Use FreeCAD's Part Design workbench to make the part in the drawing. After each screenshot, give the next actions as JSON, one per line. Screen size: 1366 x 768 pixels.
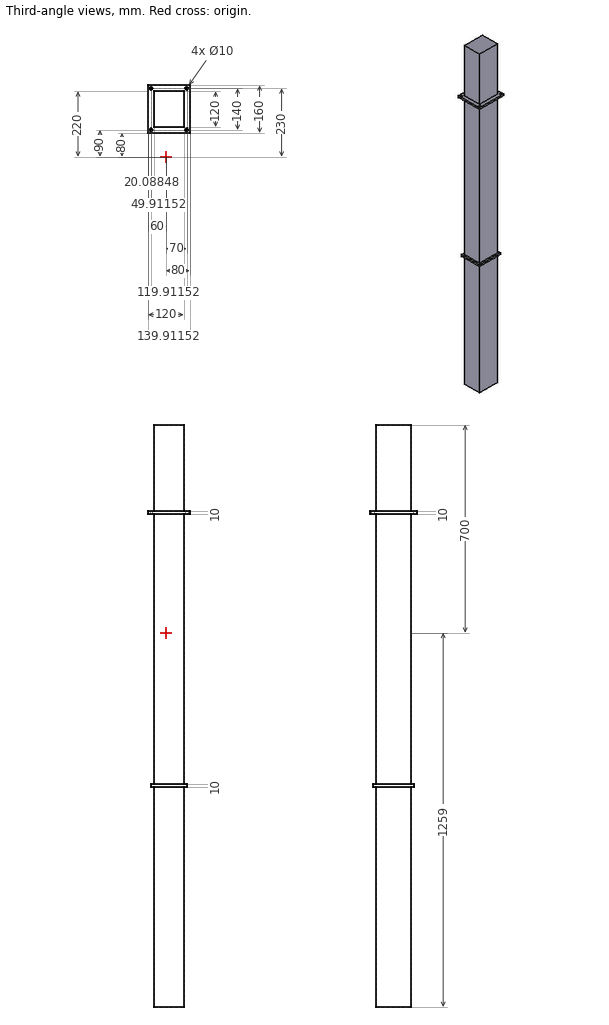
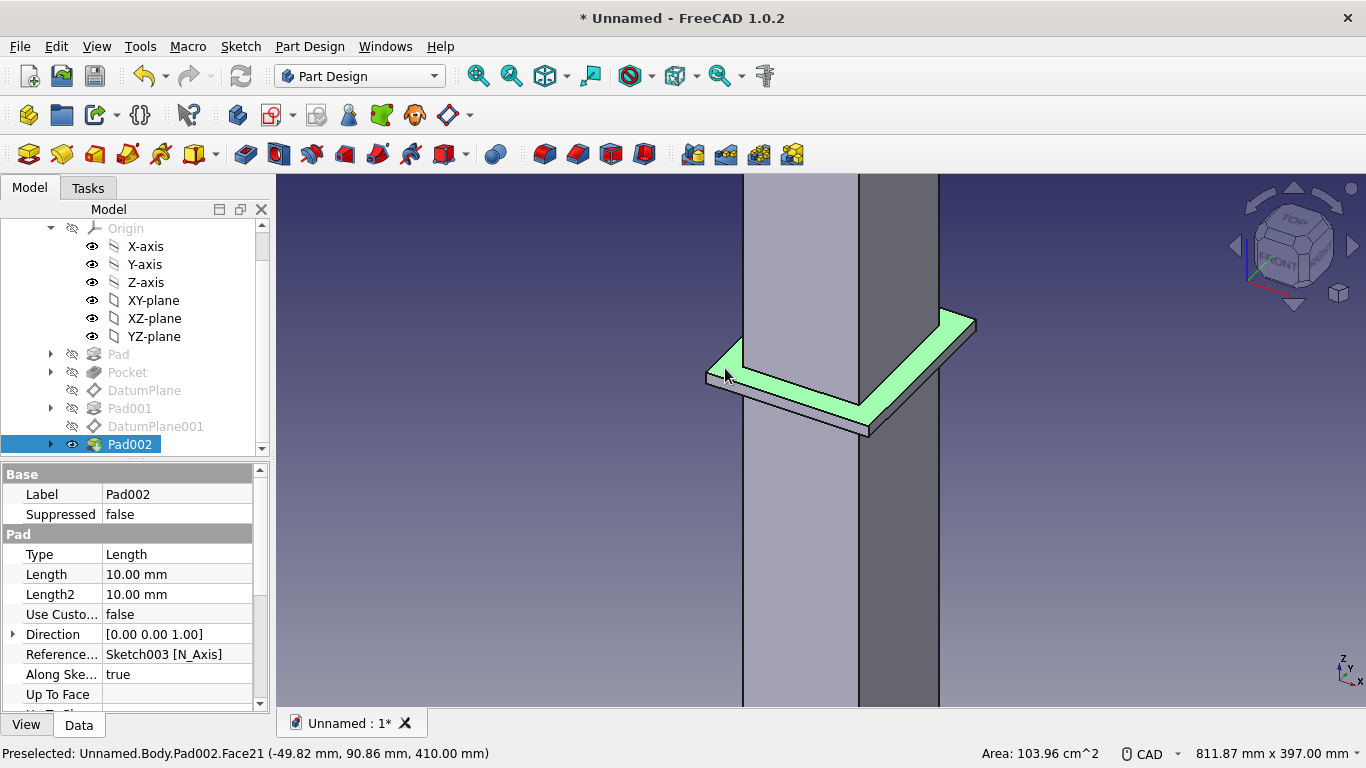
{"action": "left_click", "coordinate": [270, 116]}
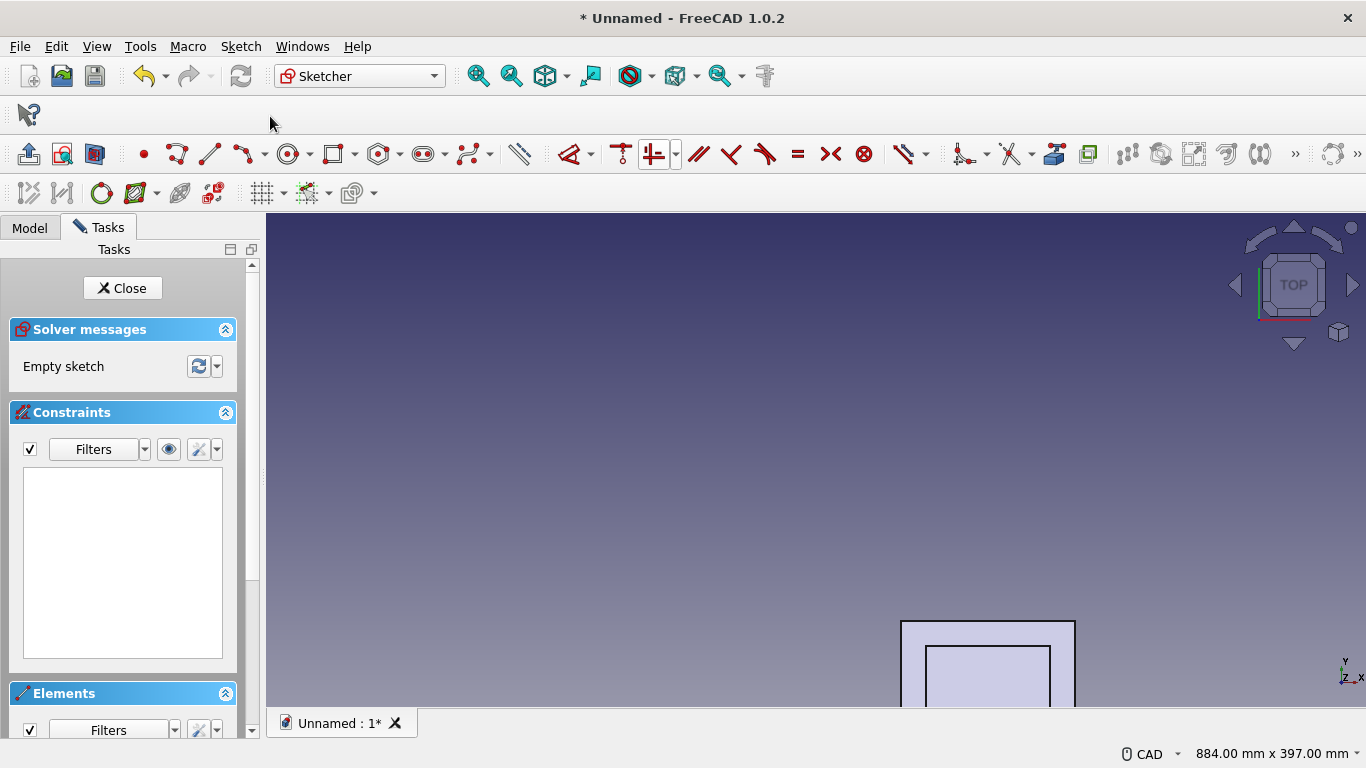
{"action": "key", "text": "q s"}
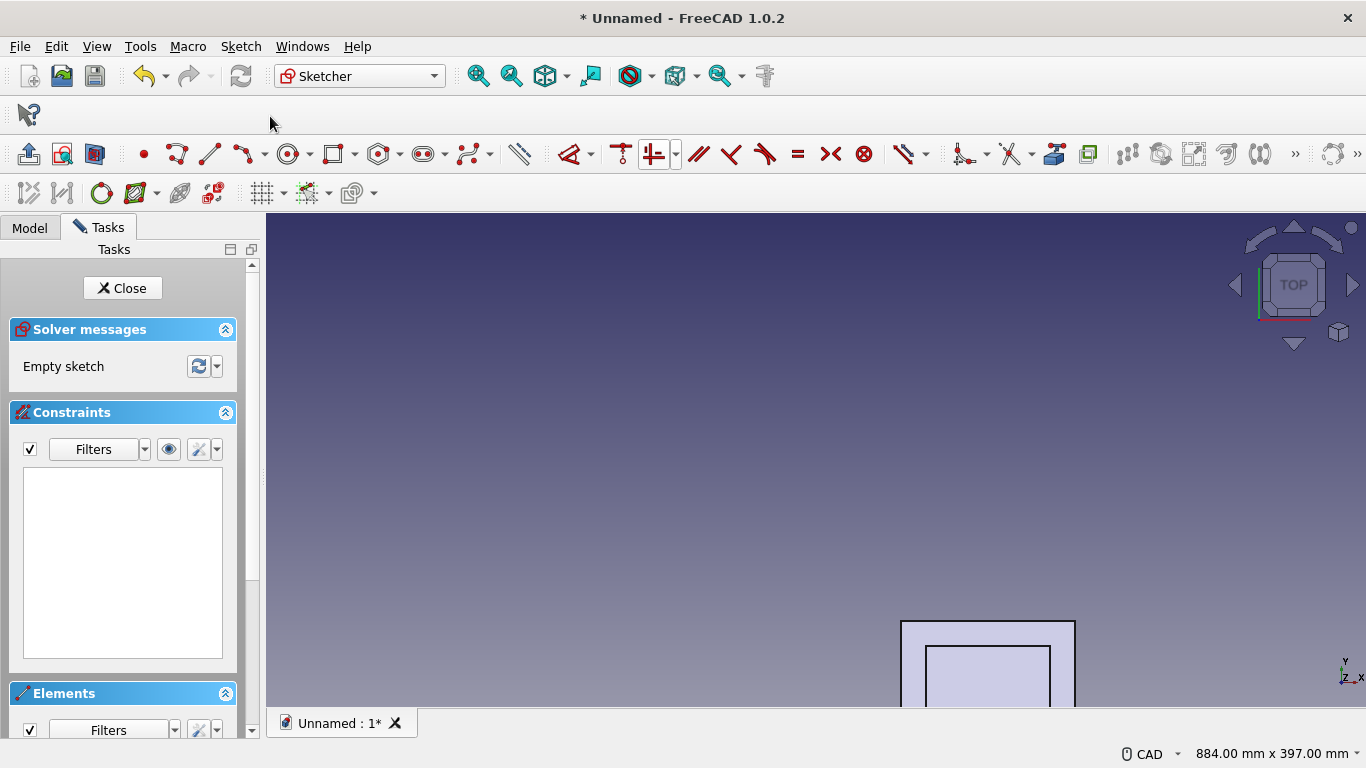
{"action": "scroll", "coordinate": [455, 241], "scroll_direction": "down", "scroll_amount": 3}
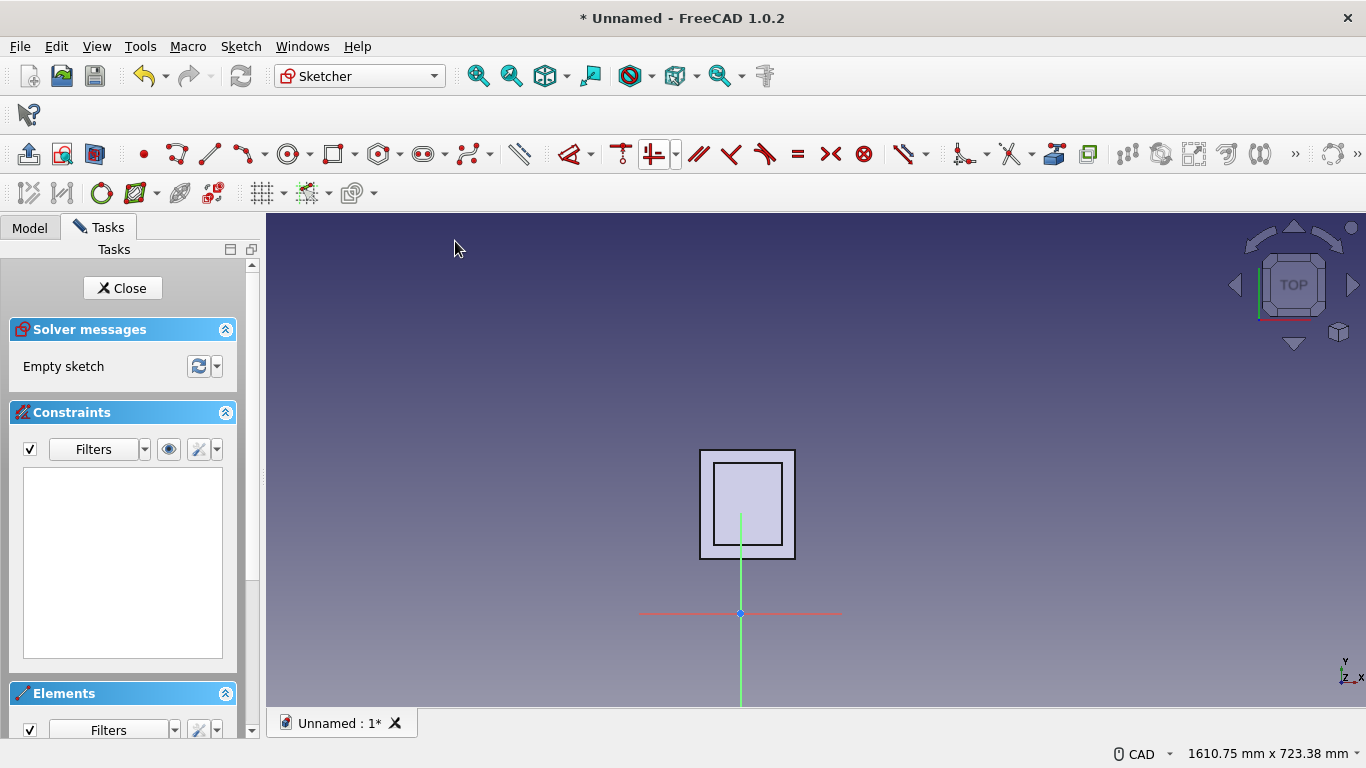
{"action": "scroll", "coordinate": [748, 623], "scroll_direction": "up", "scroll_amount": 3}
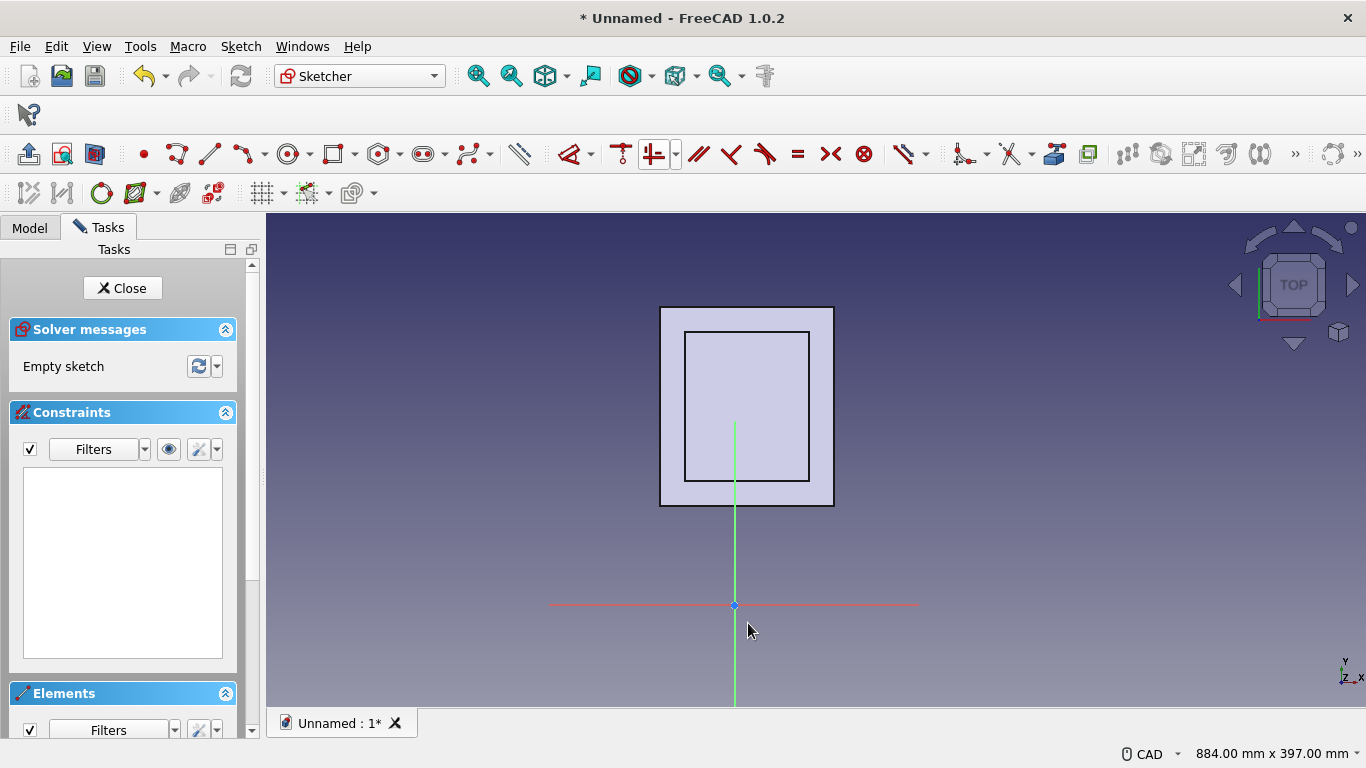
{"action": "key", "text": "g c"}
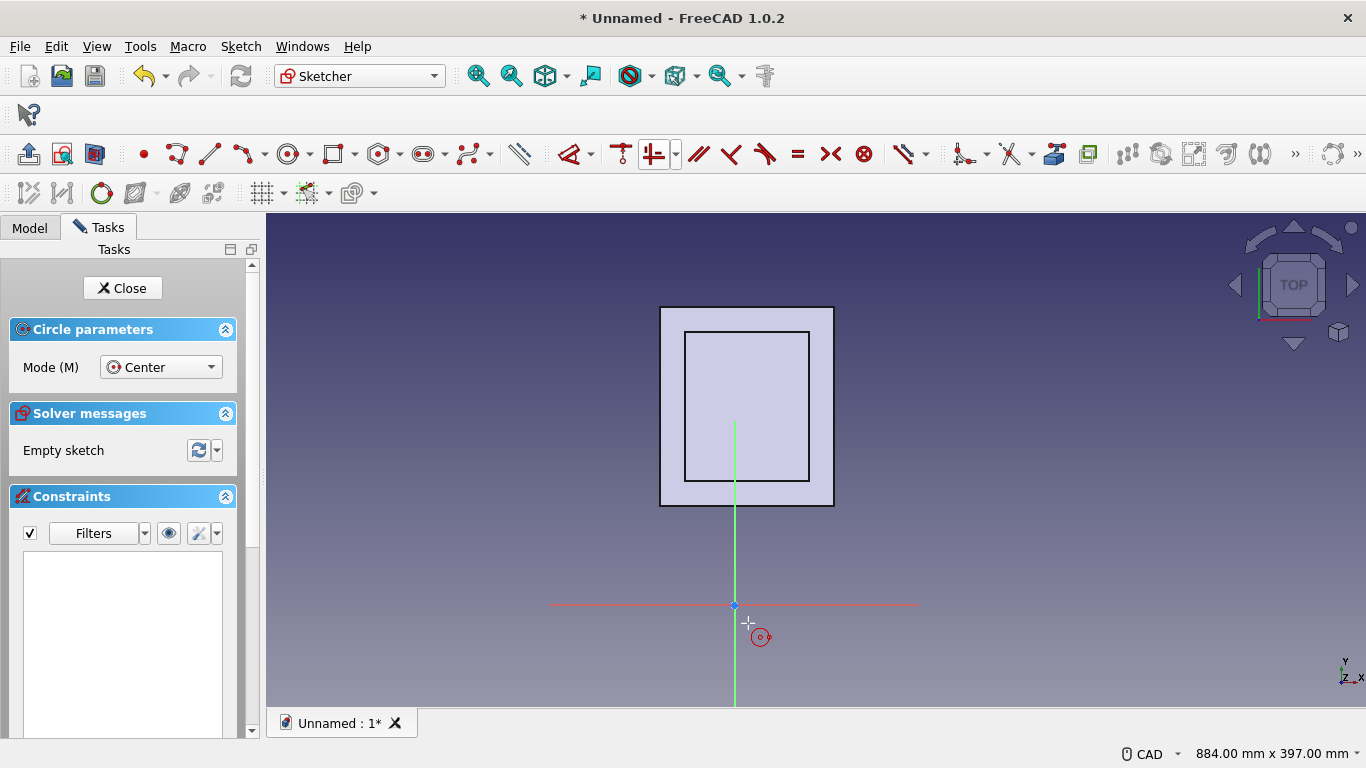
{"action": "scroll", "coordinate": [822, 319], "scroll_direction": "up", "scroll_amount": 7}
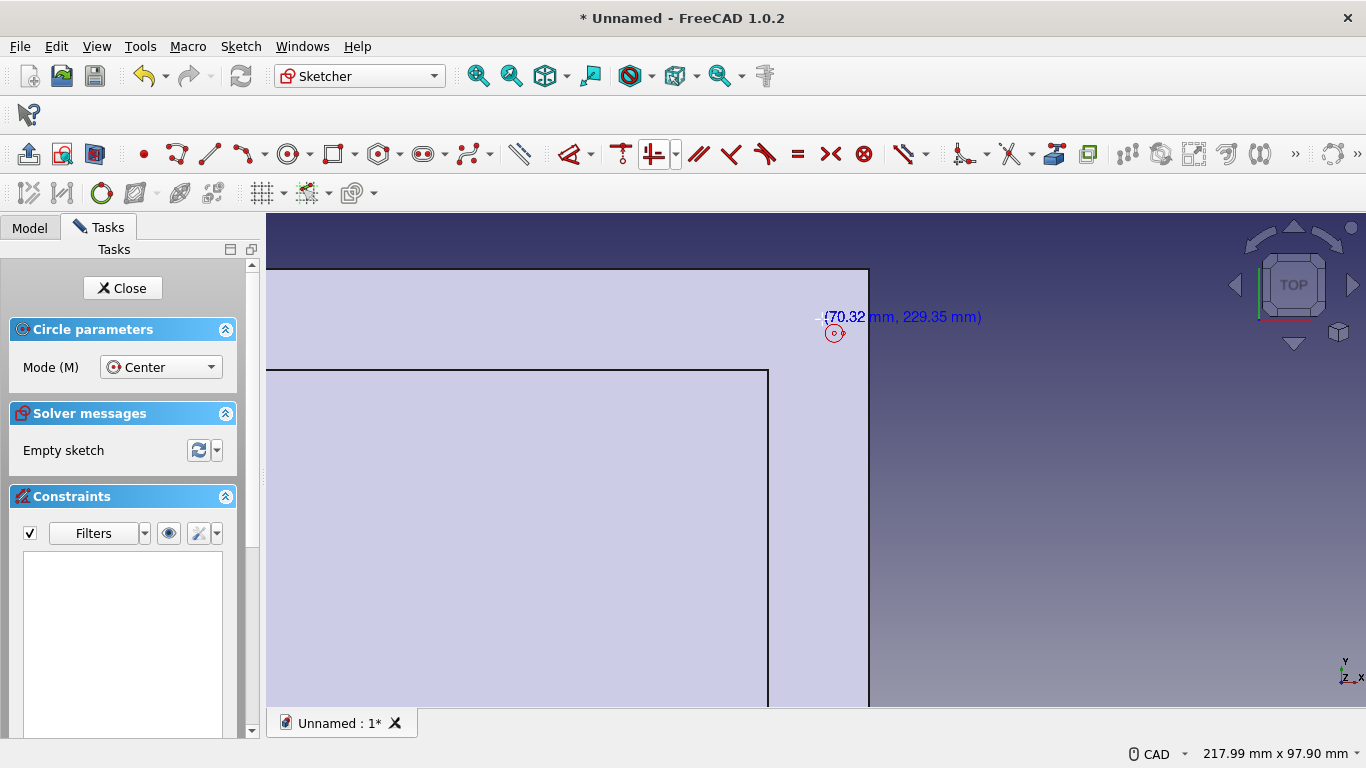
{"action": "scroll", "coordinate": [823, 320], "scroll_direction": "down", "scroll_amount": 7}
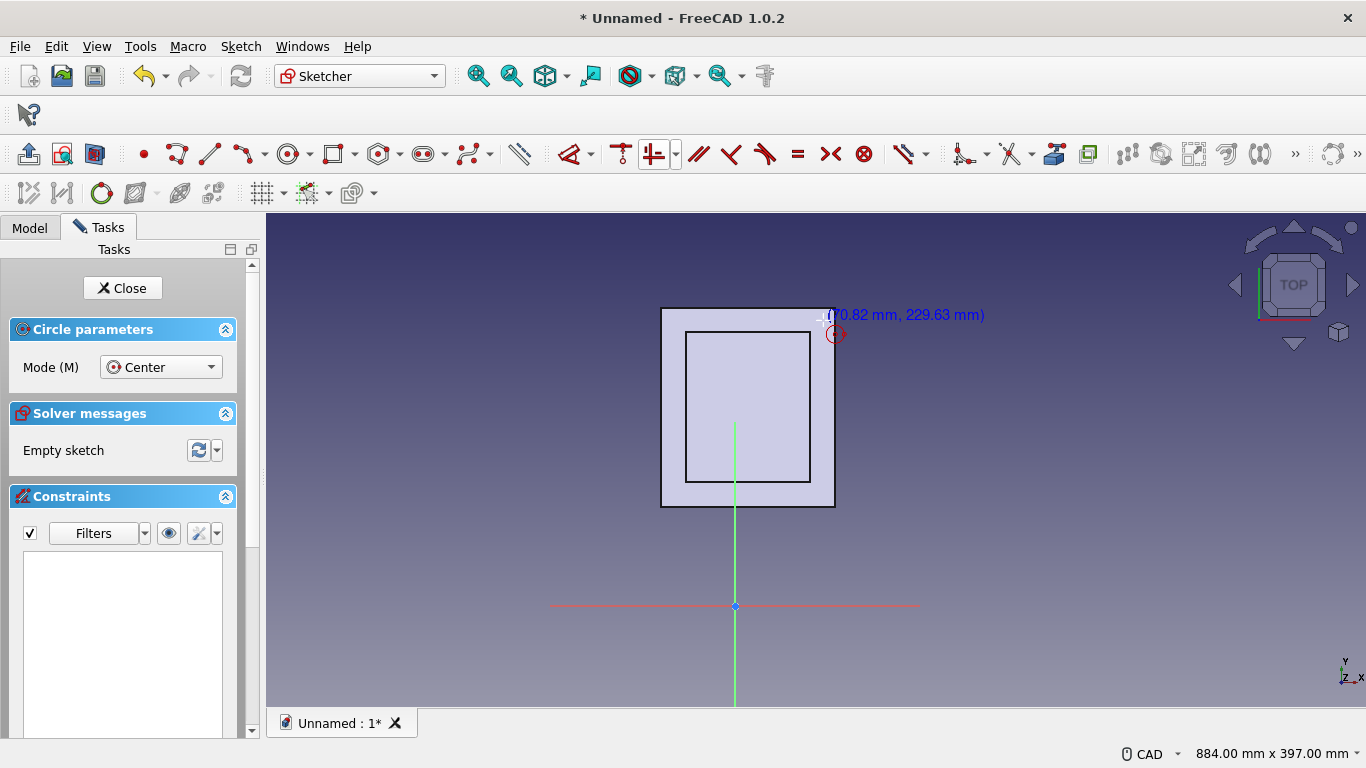
{"action": "left_click", "coordinate": [822, 320]}
{"action": "mouse_move", "coordinate": [827, 316]}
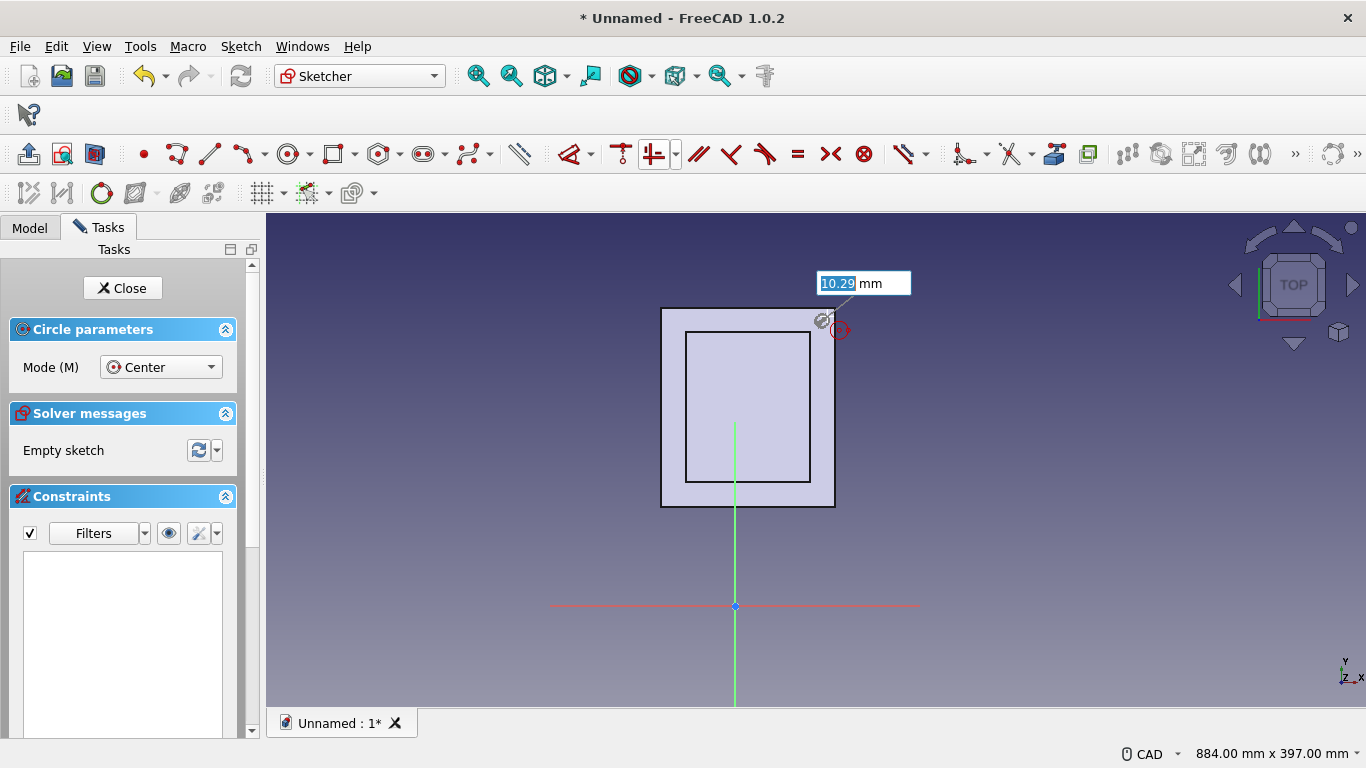
{"action": "type", "text": "10"}
{"action": "key", "text": "Return"}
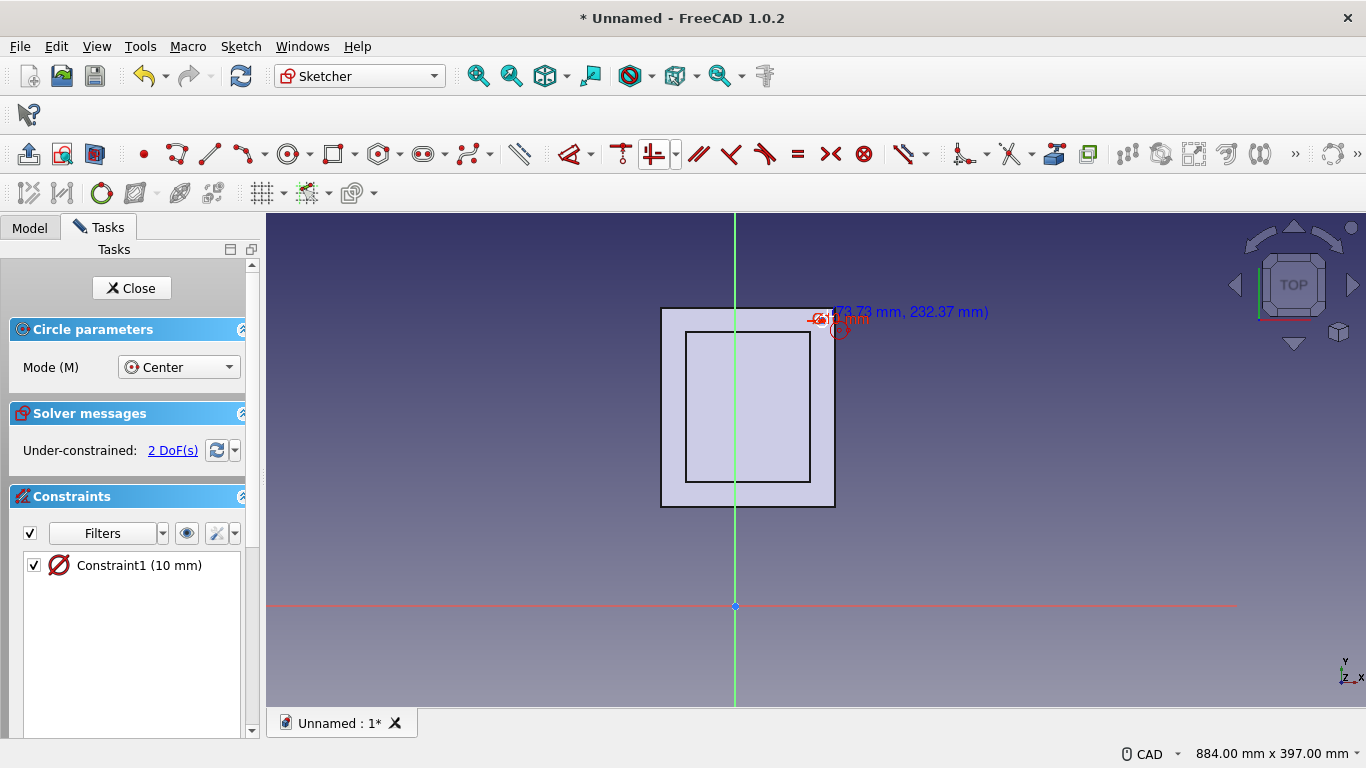
{"action": "scroll", "coordinate": [822, 494], "scroll_direction": "up", "scroll_amount": 7}